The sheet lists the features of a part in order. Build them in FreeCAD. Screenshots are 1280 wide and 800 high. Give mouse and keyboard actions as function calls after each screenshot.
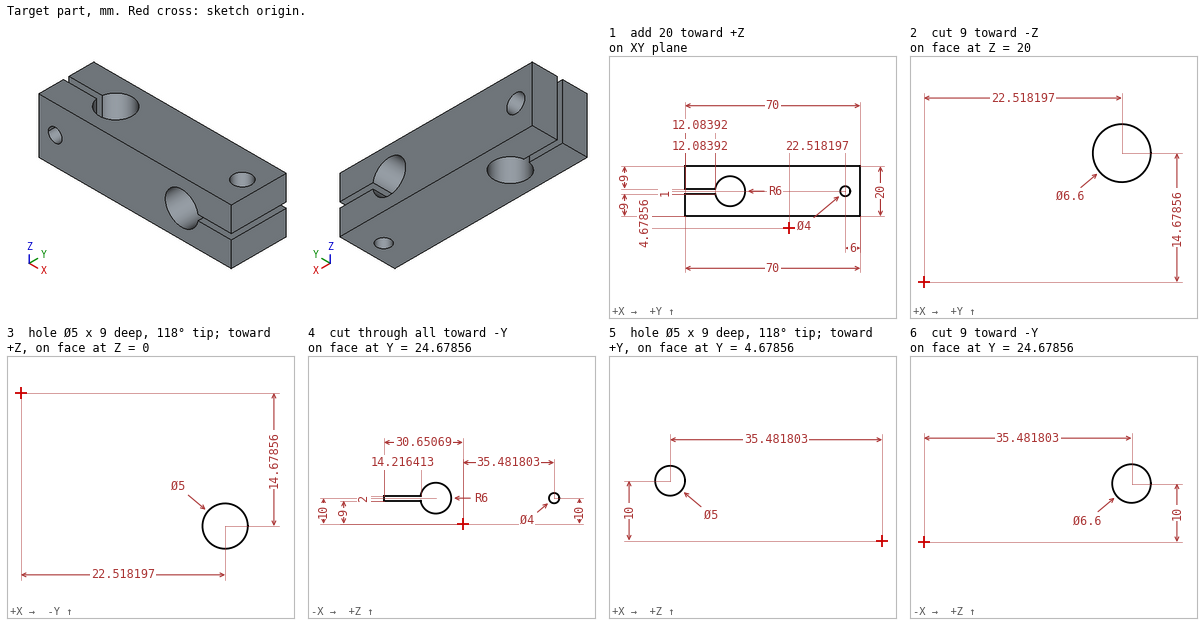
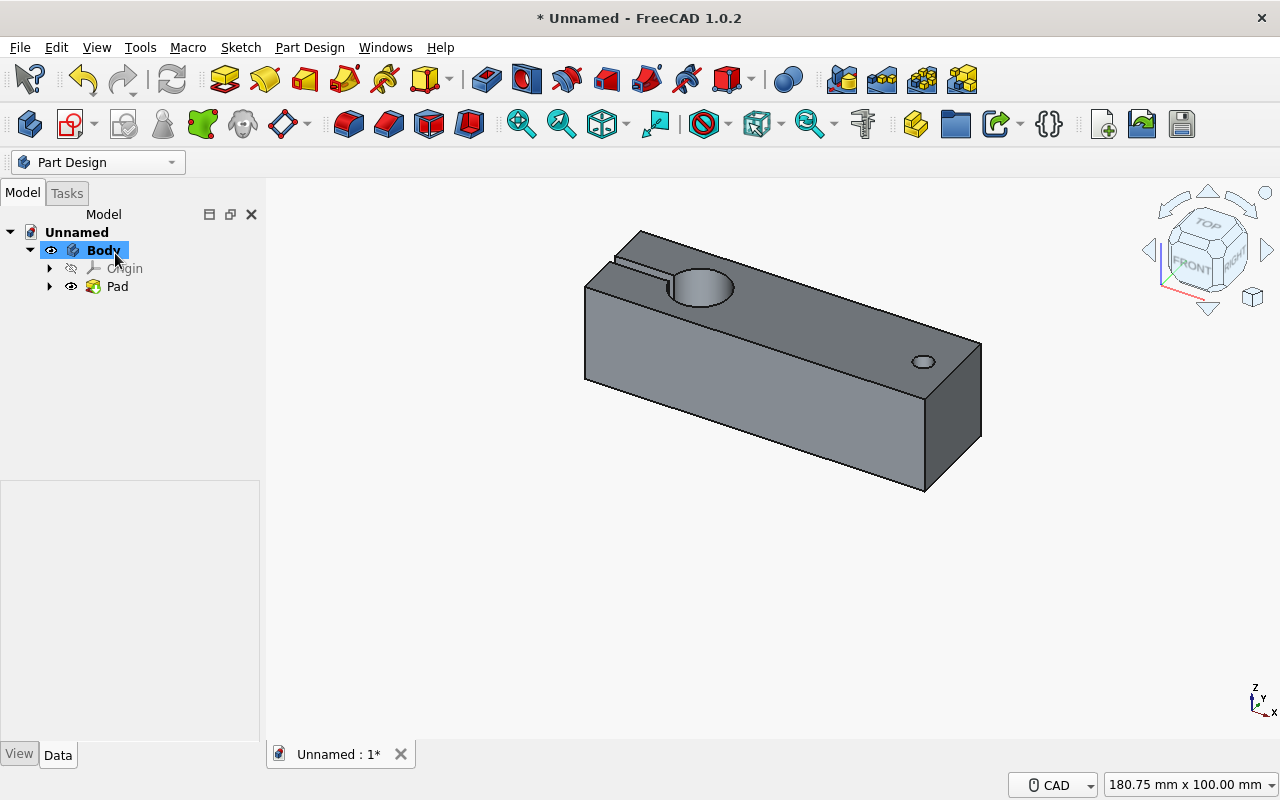
click(831, 330)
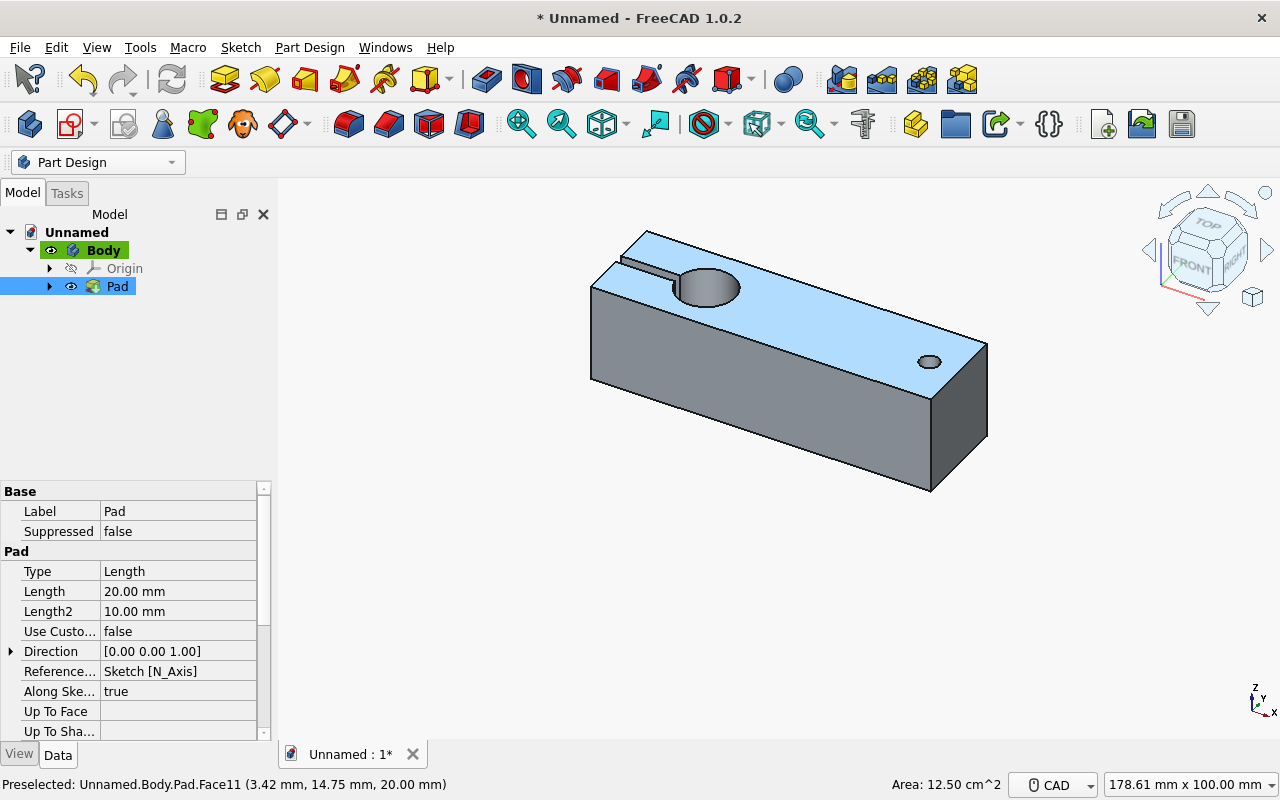
click(70, 124)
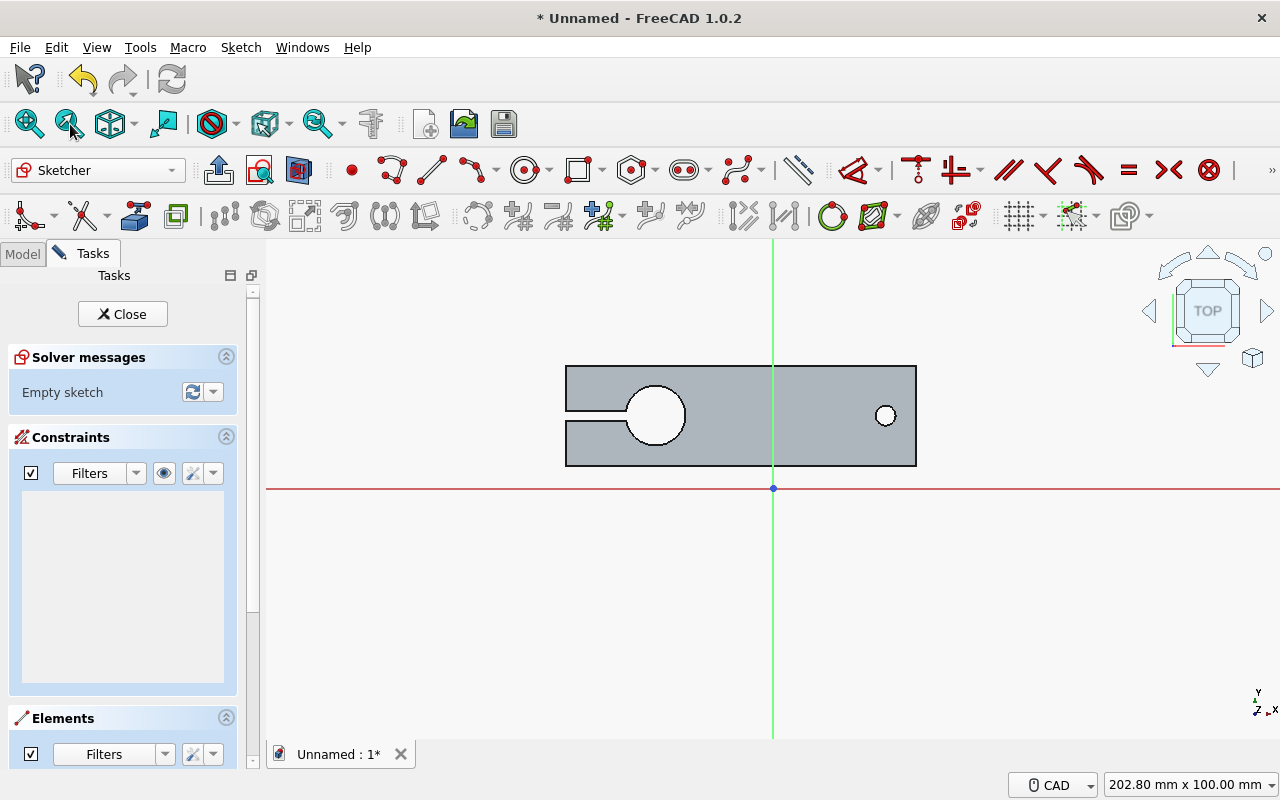
scroll(908, 406, up, 11)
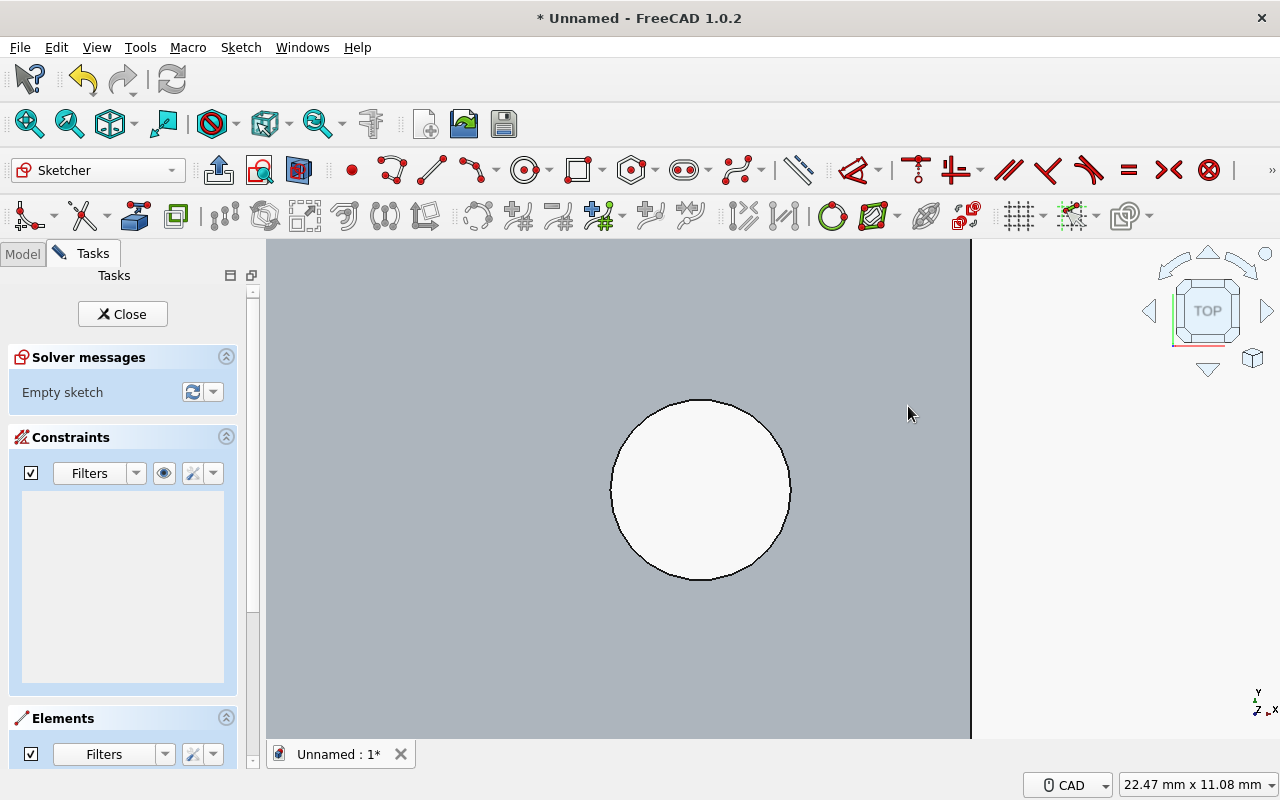
click(526, 170)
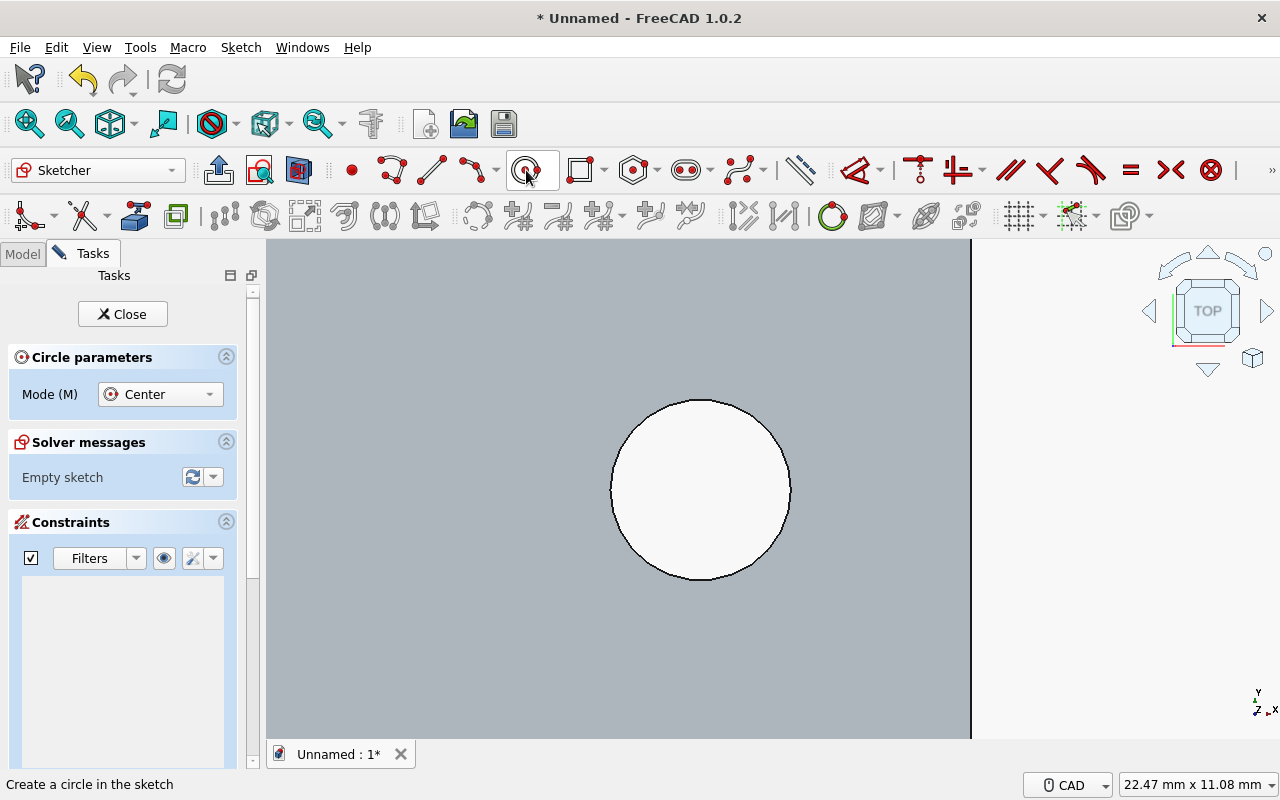
click(701, 490)
click(806, 385)
key(Escape)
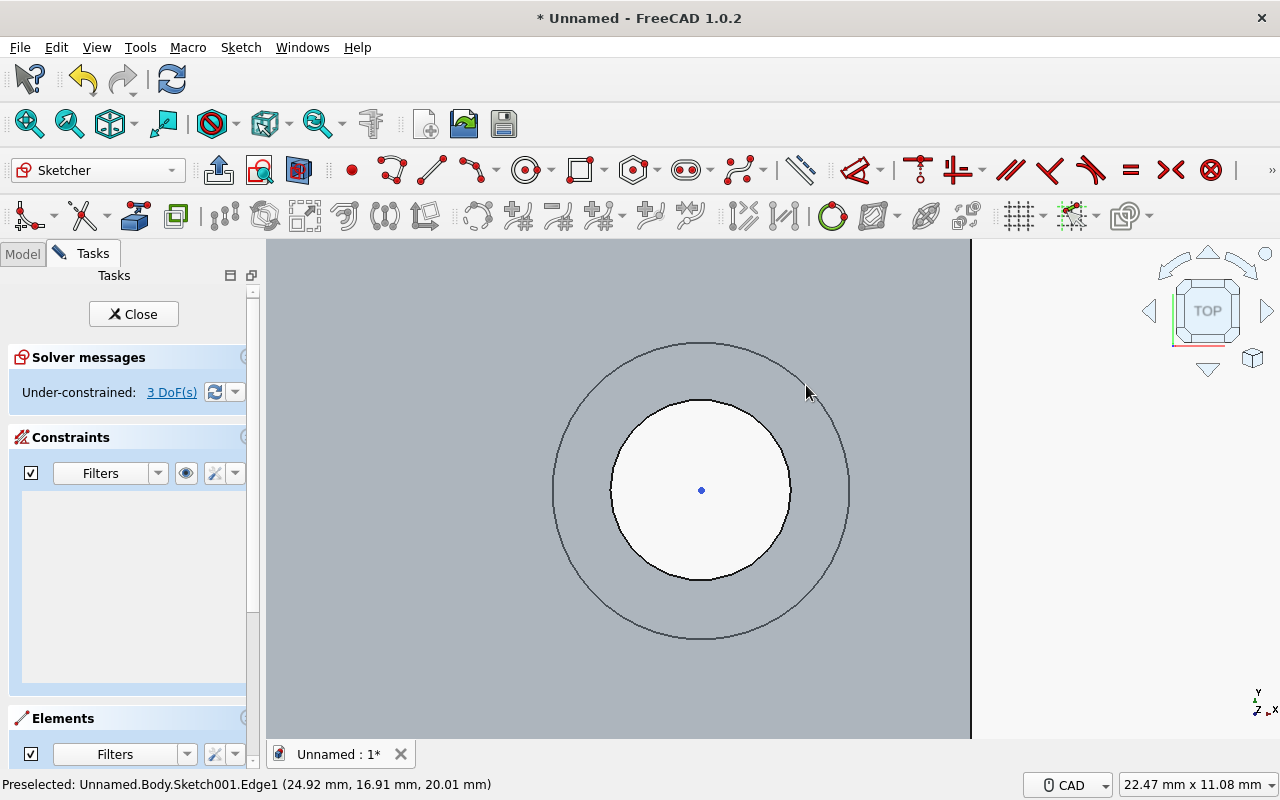
click(856, 170)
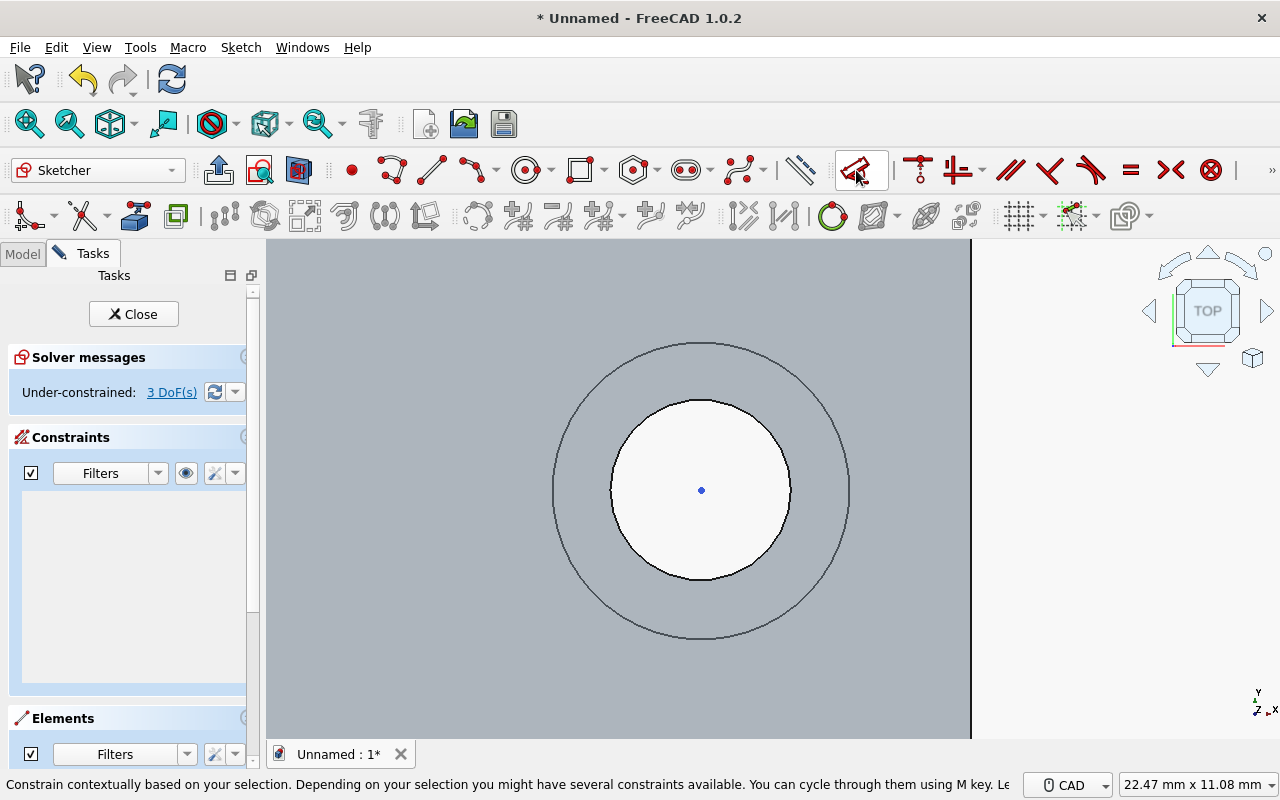
click(806, 386)
click(829, 363)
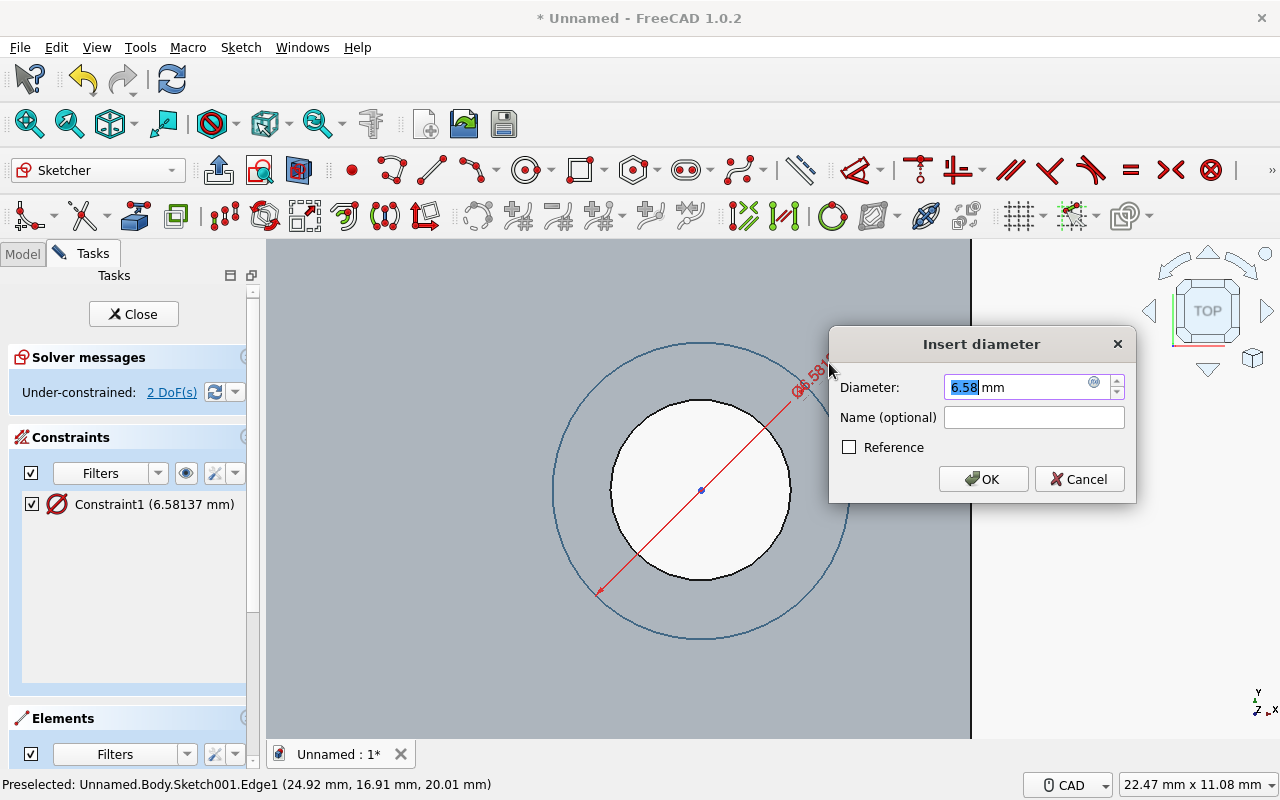
text(6.6)
key(Return)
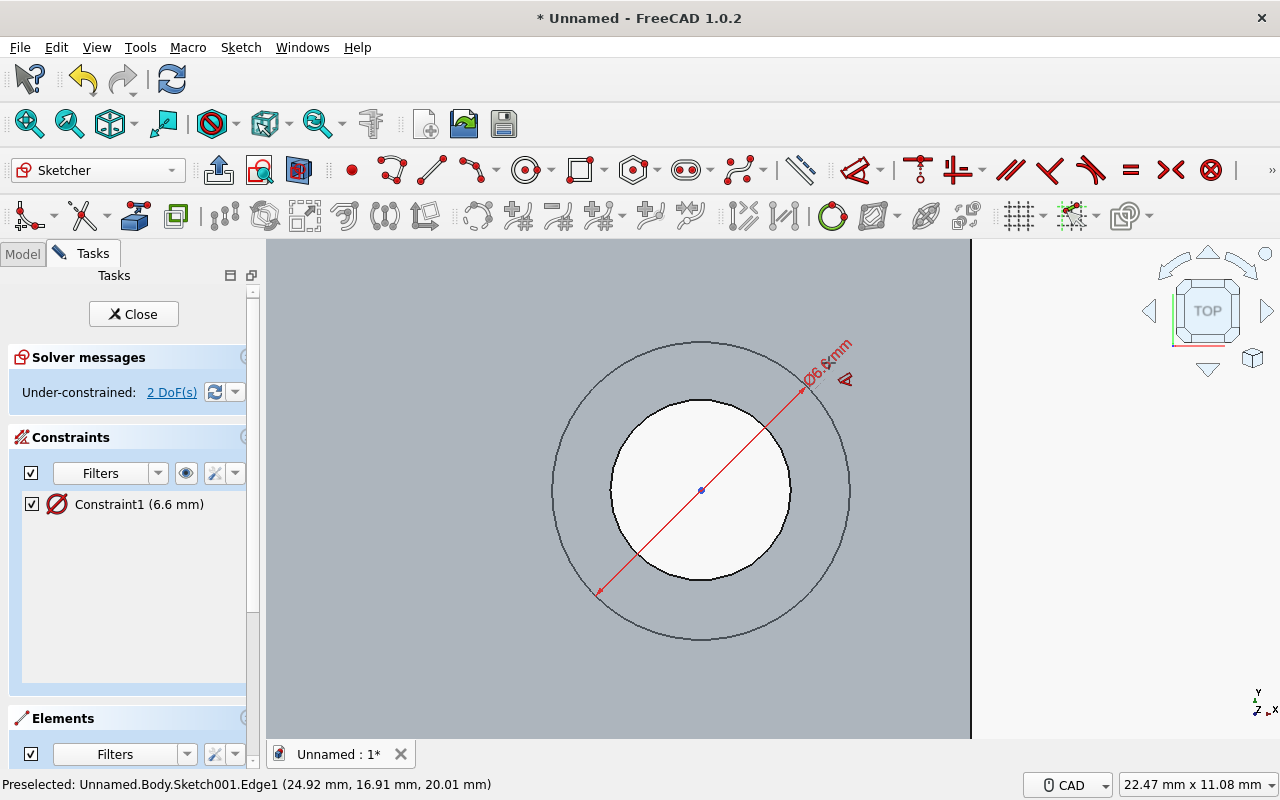
click(701, 491)
click(735, 601)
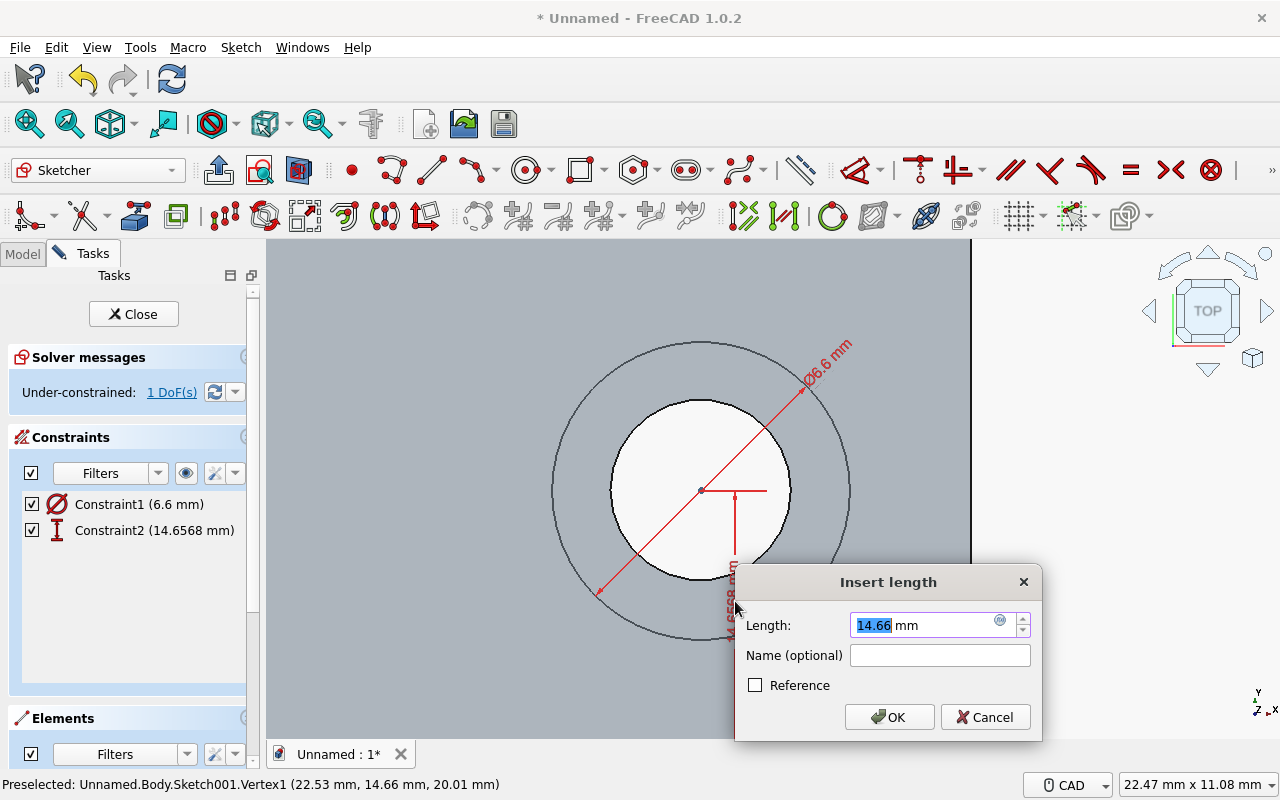
text(14.67856)
key(Return)